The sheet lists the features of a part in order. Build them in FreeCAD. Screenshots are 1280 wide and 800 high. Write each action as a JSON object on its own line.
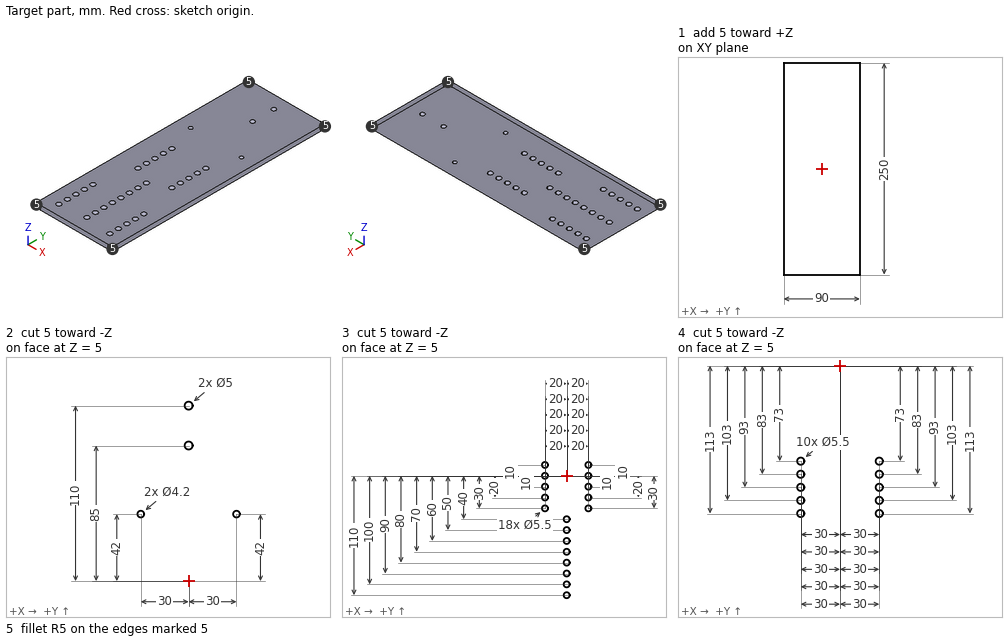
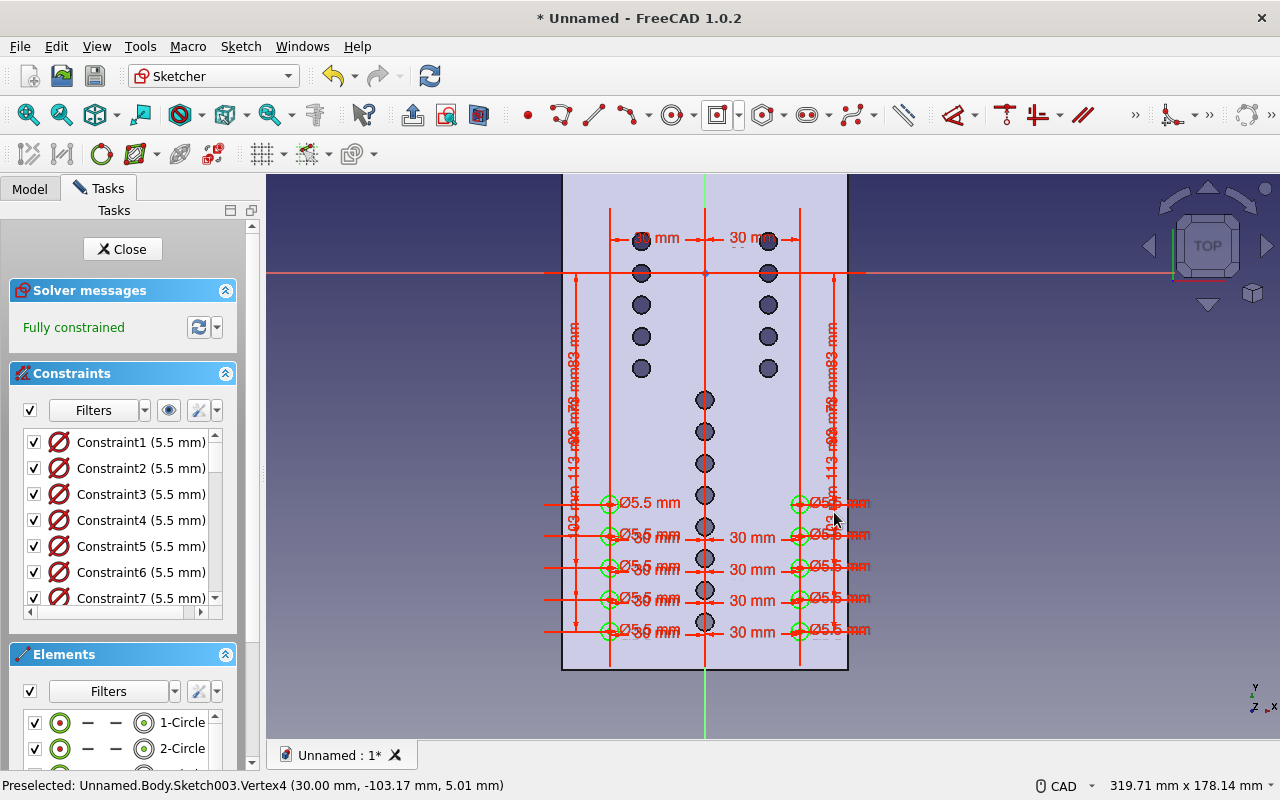
{"action": "left_click", "coordinate": [123, 249]}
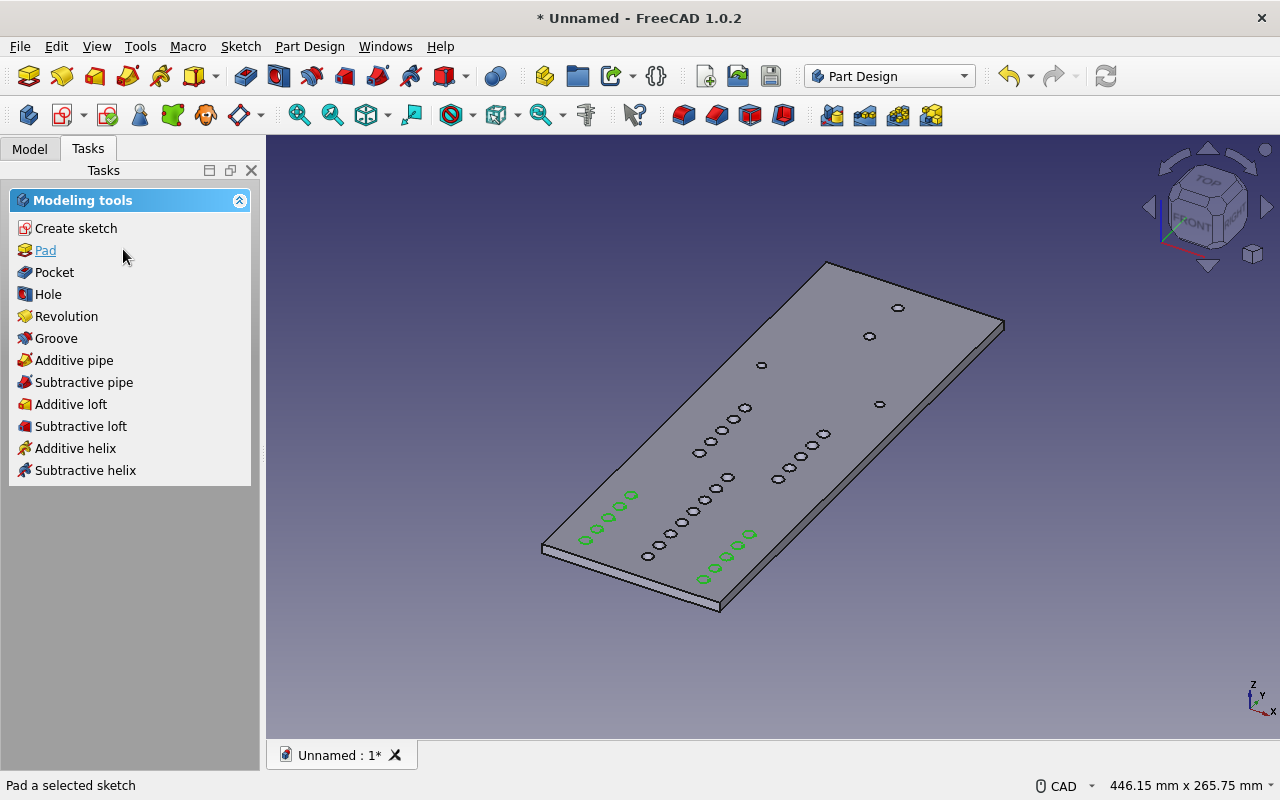
{"action": "left_click", "coordinate": [246, 76]}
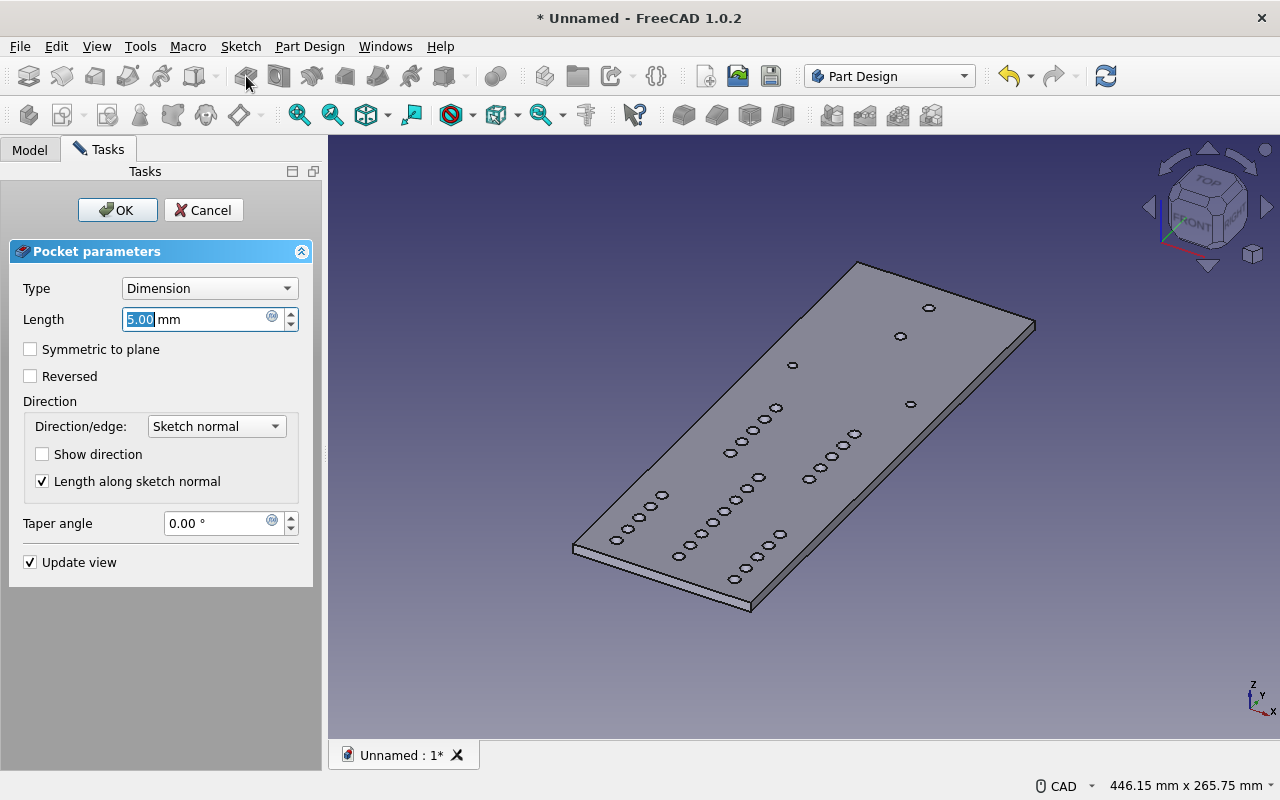
{"action": "type", "text": "5"}
{"action": "key", "text": "Tab"}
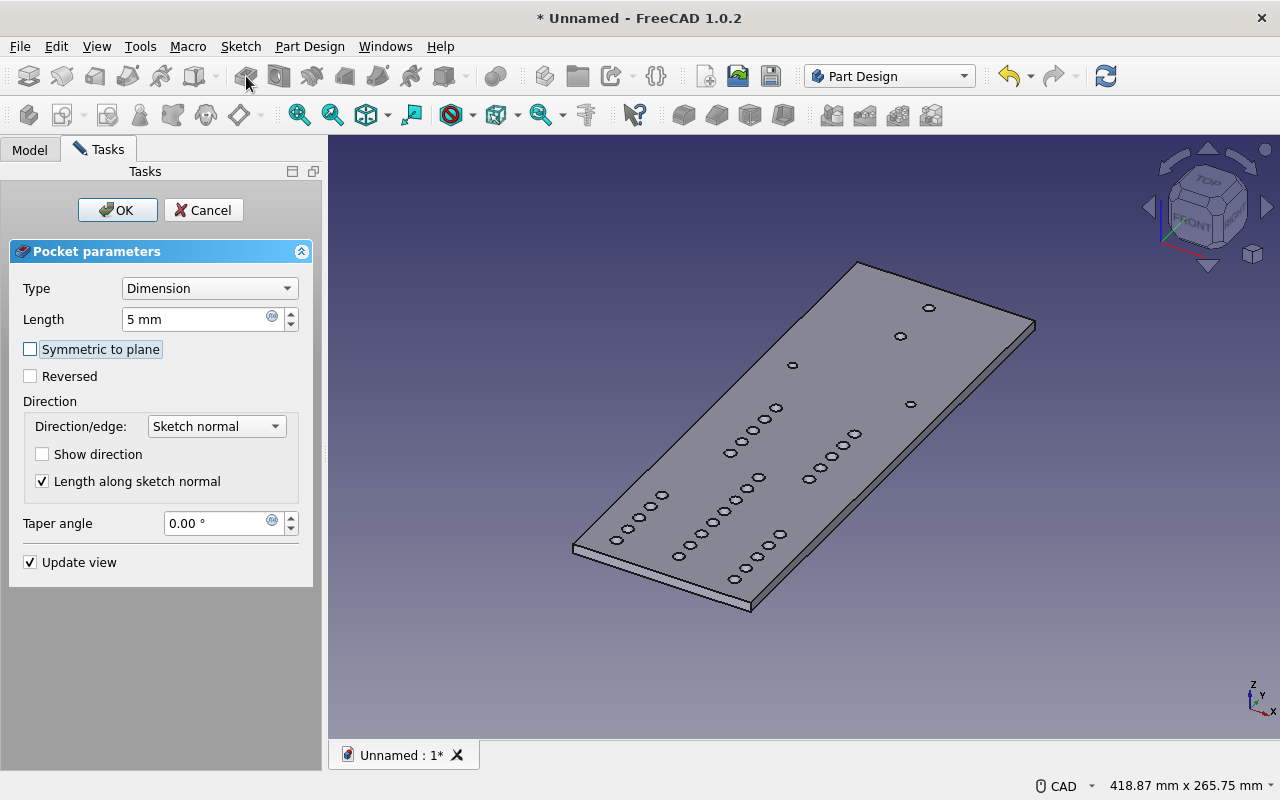
{"action": "left_click", "coordinate": [118, 210]}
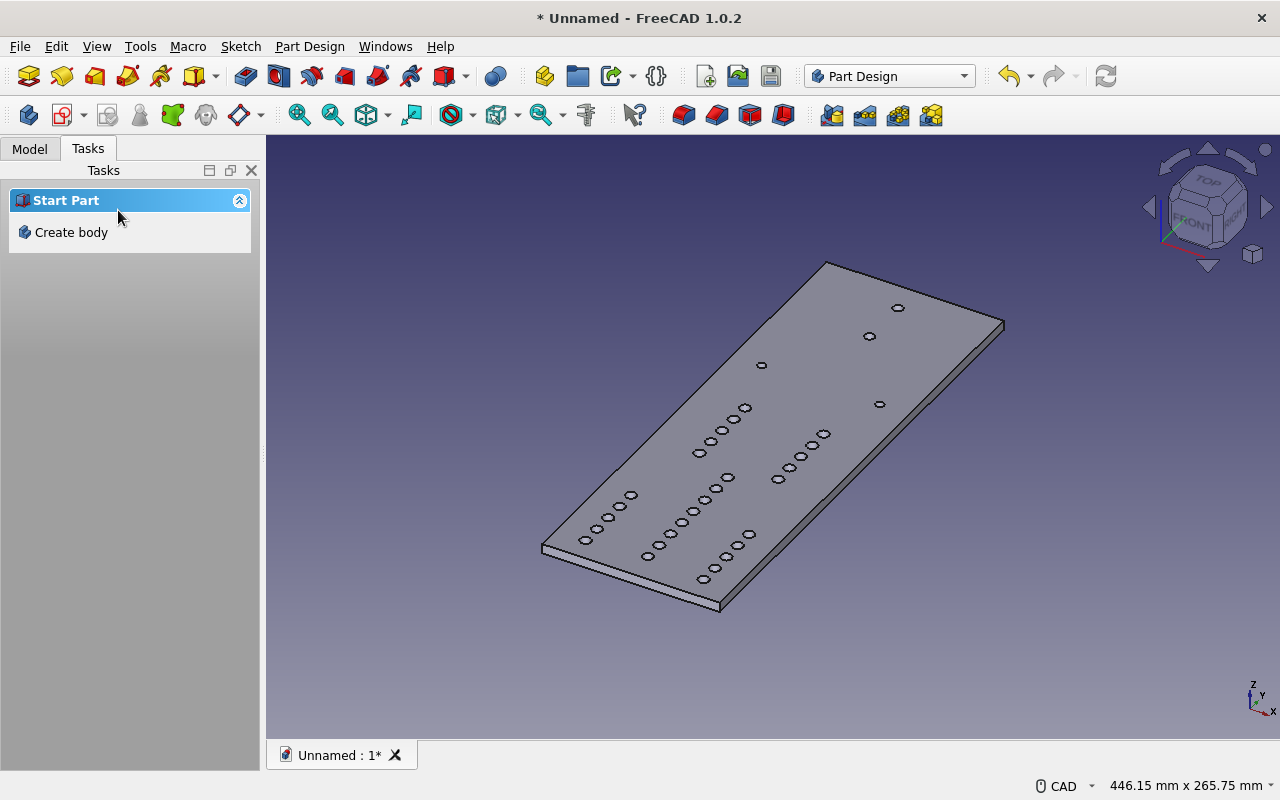
{"action": "left_click", "coordinate": [720, 608]}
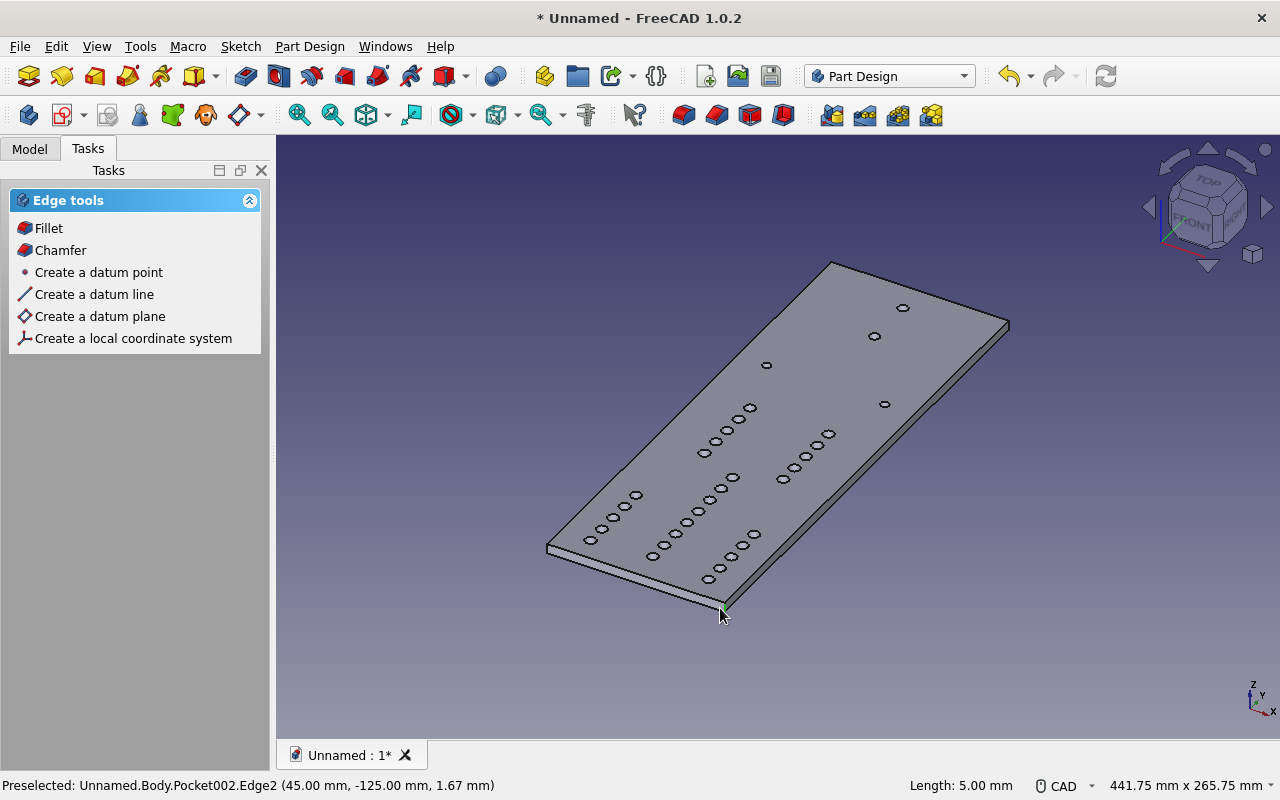
{"action": "scroll", "coordinate": [547, 548], "scroll_direction": "up", "scroll_amount": 7}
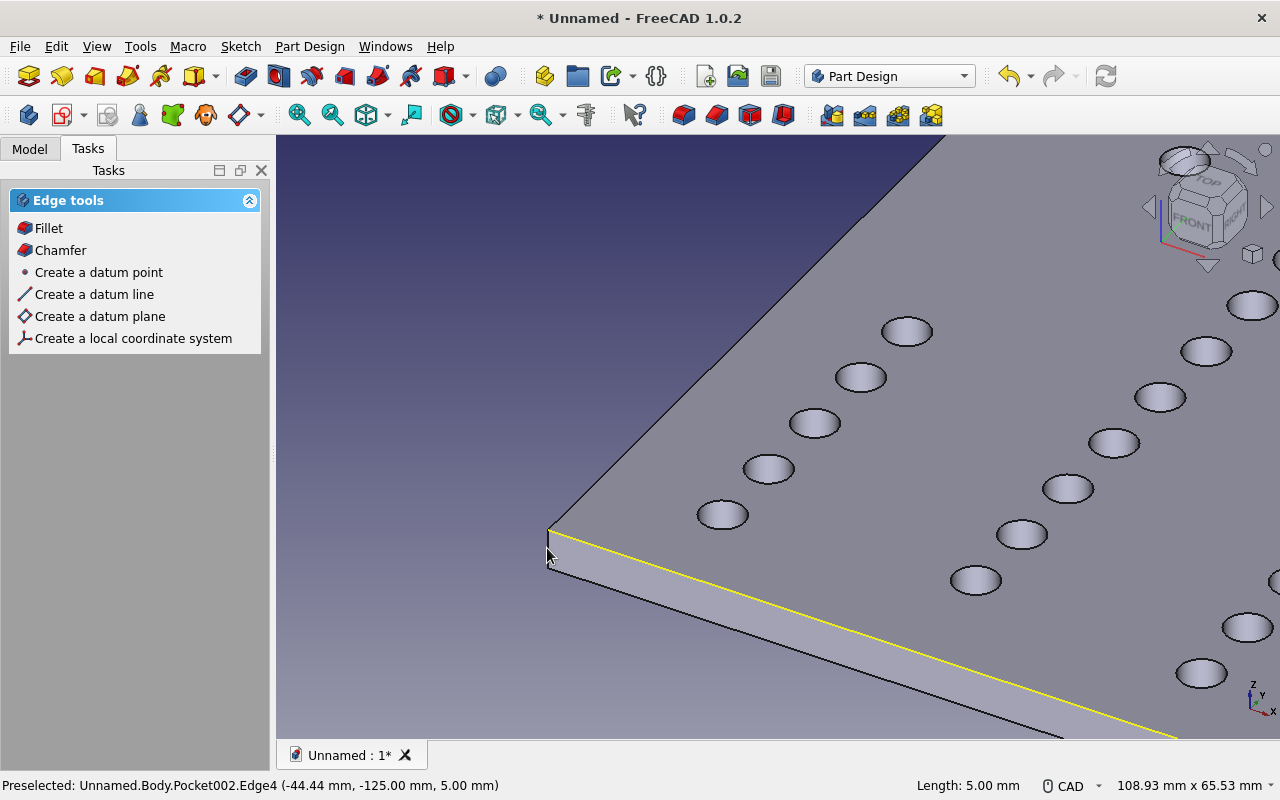
{"action": "key", "text": "v f"}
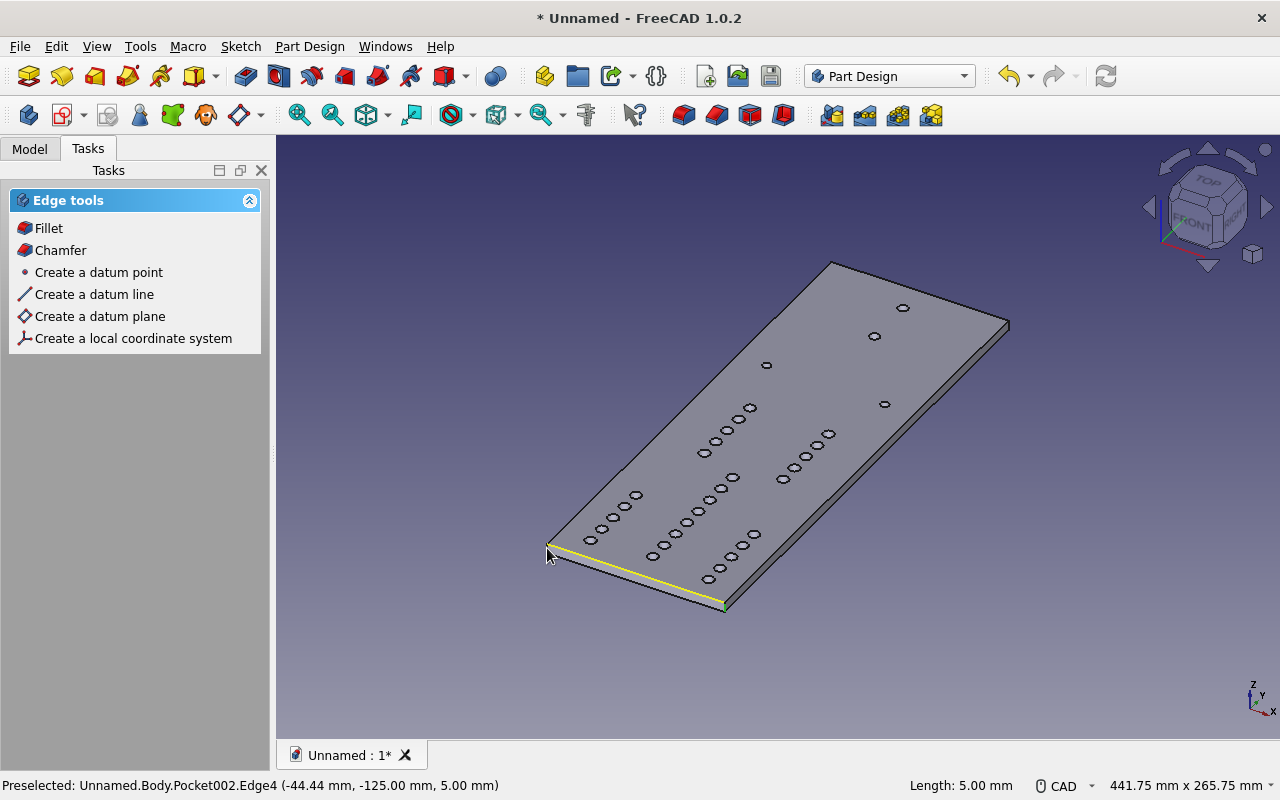
{"action": "key", "text": "0"}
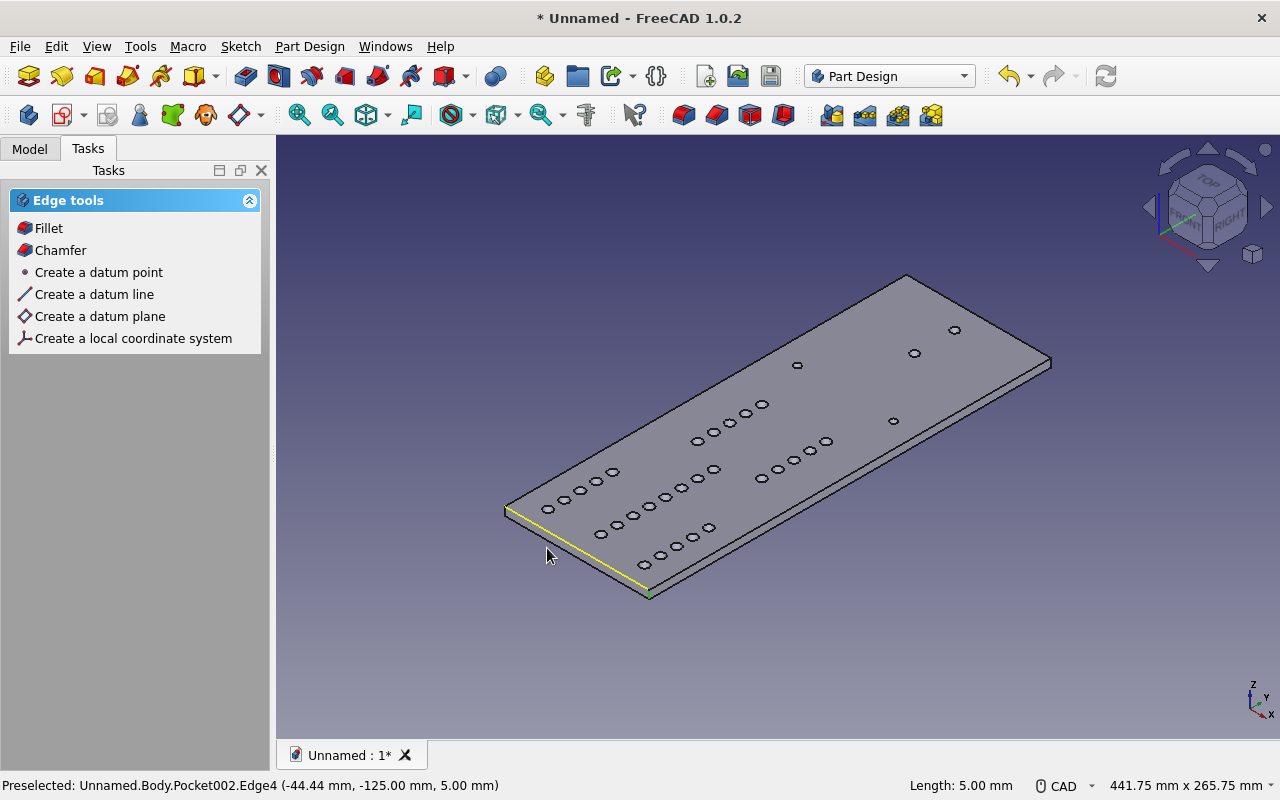
{"action": "scroll", "coordinate": [505, 510], "scroll_direction": "up", "scroll_amount": 7}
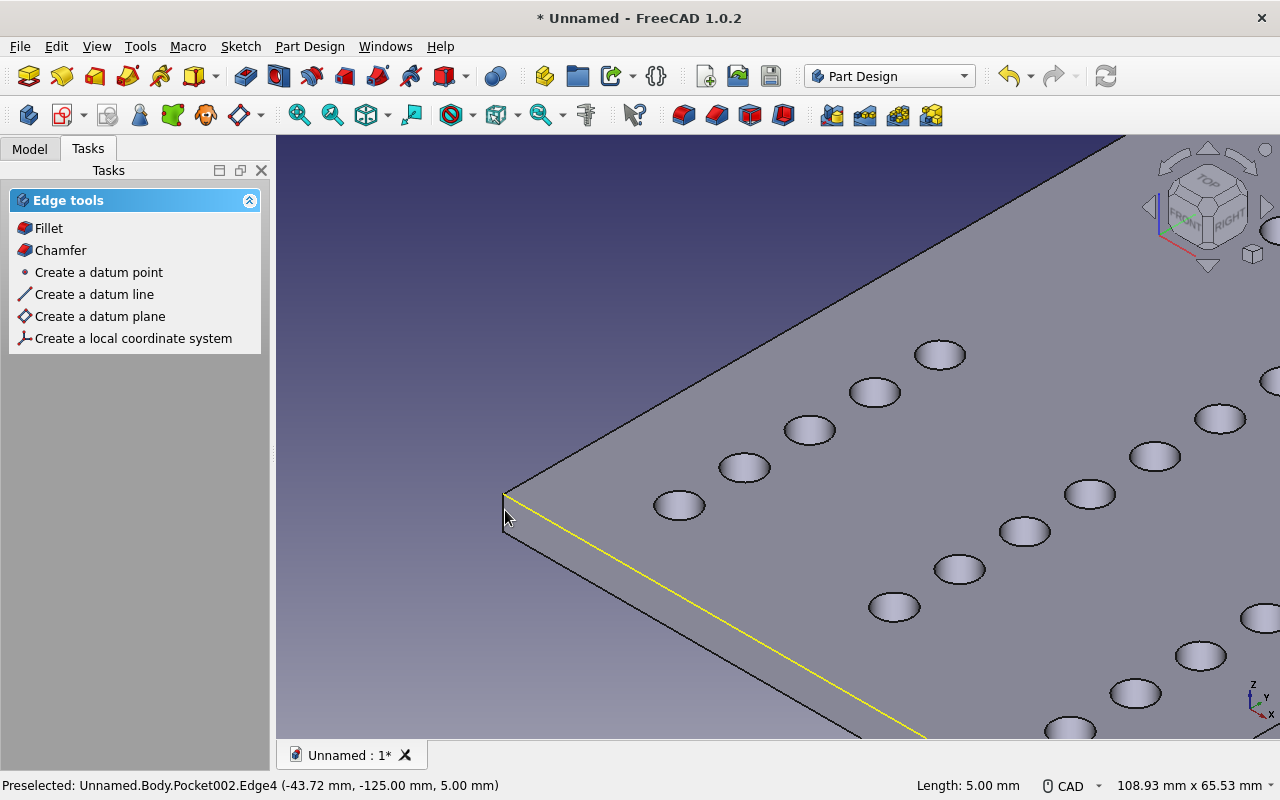
{"action": "key", "text": "v f"}